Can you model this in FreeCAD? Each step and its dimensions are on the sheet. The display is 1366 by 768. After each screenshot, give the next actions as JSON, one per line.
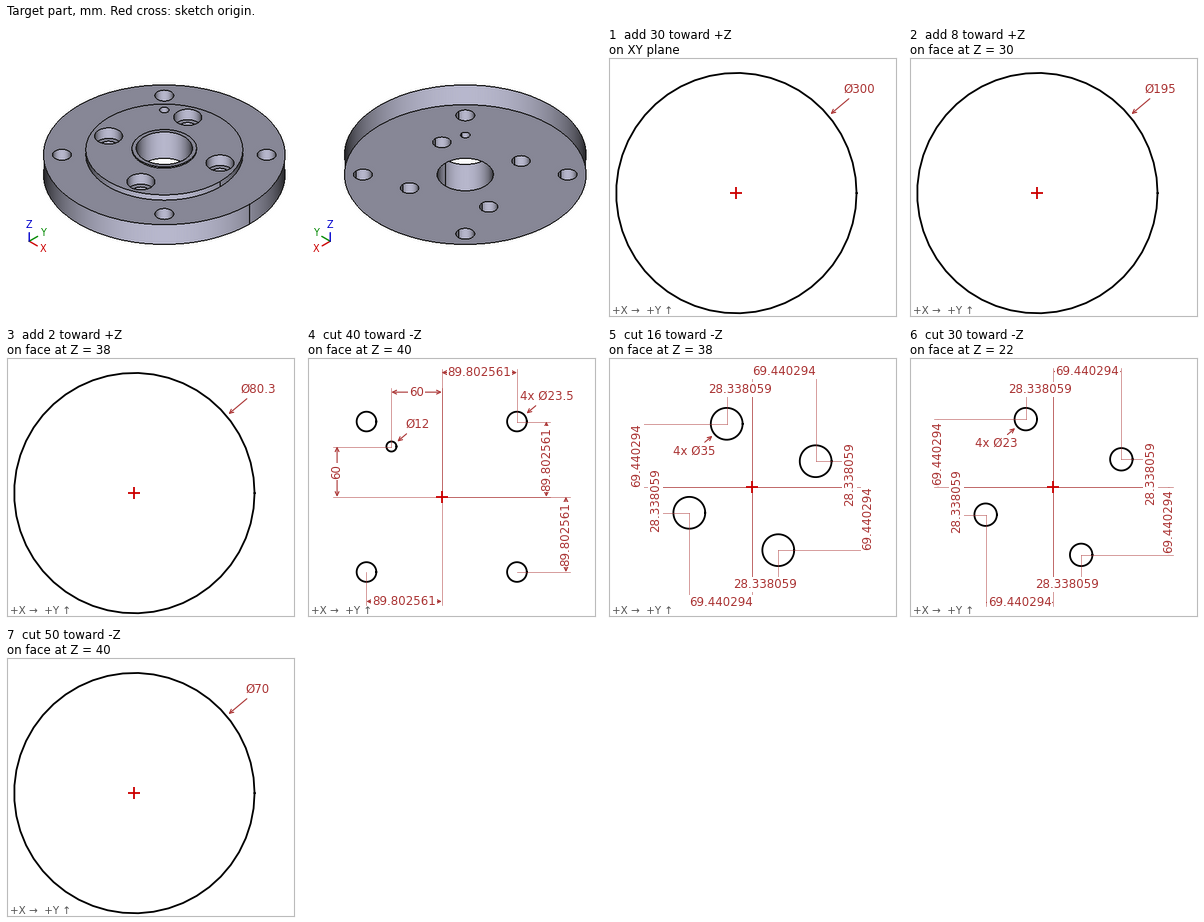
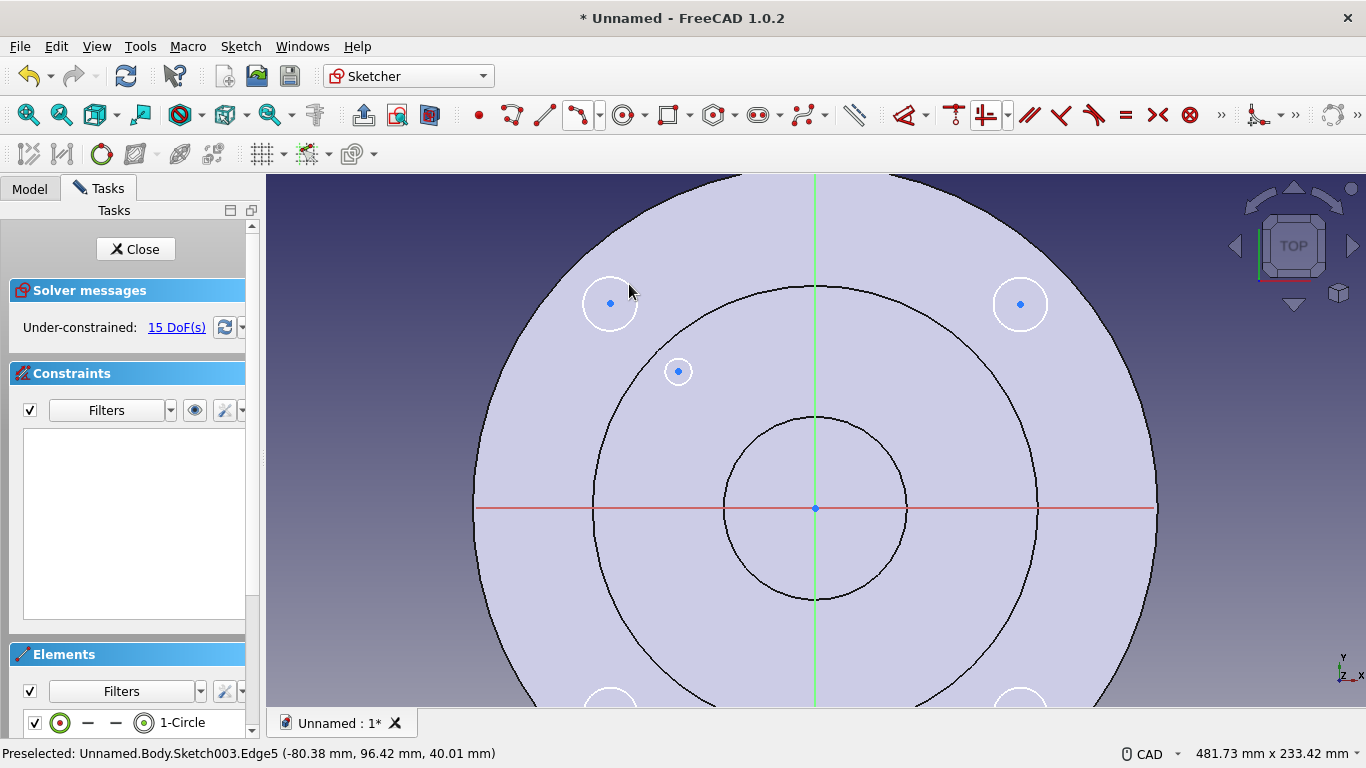
{"action": "left_click", "coordinate": [1039, 285]}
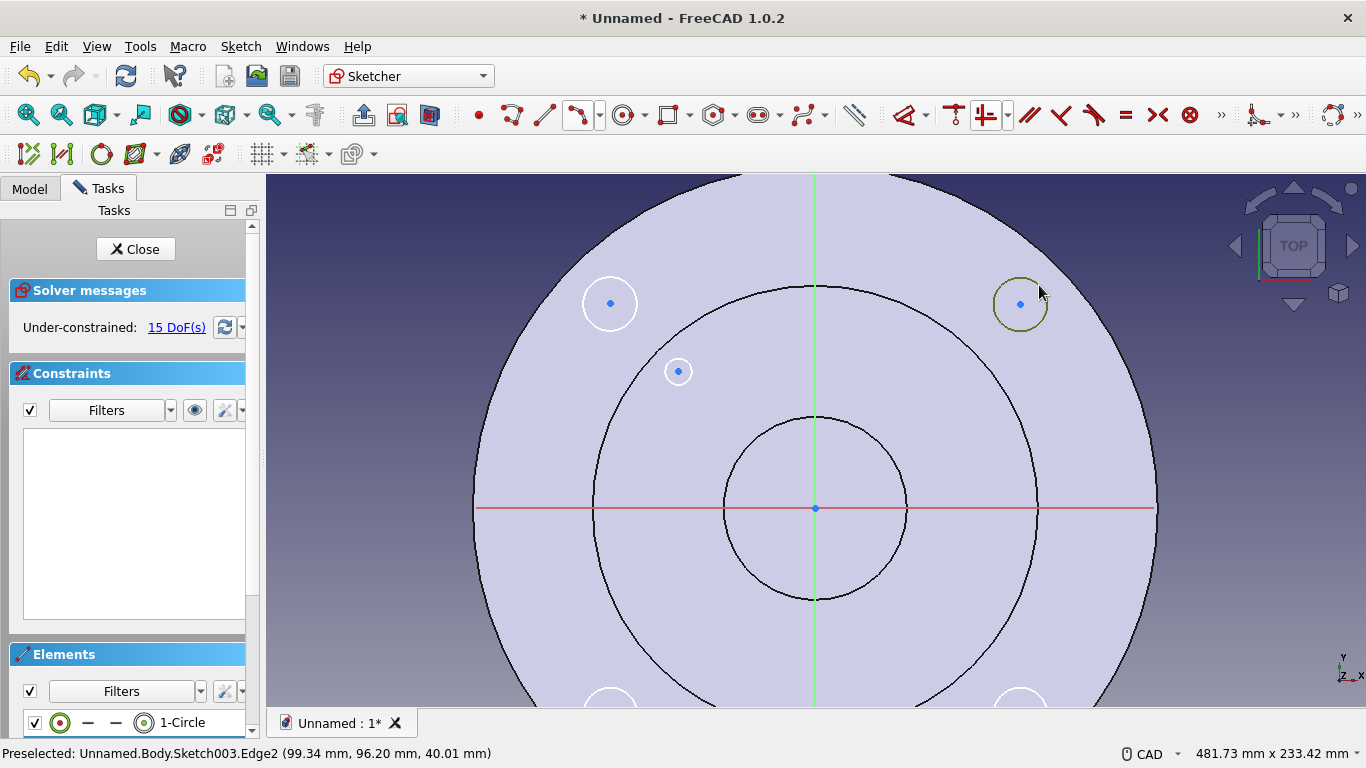
{"action": "scroll", "coordinate": [610, 303], "scroll_direction": "down", "scroll_amount": 2}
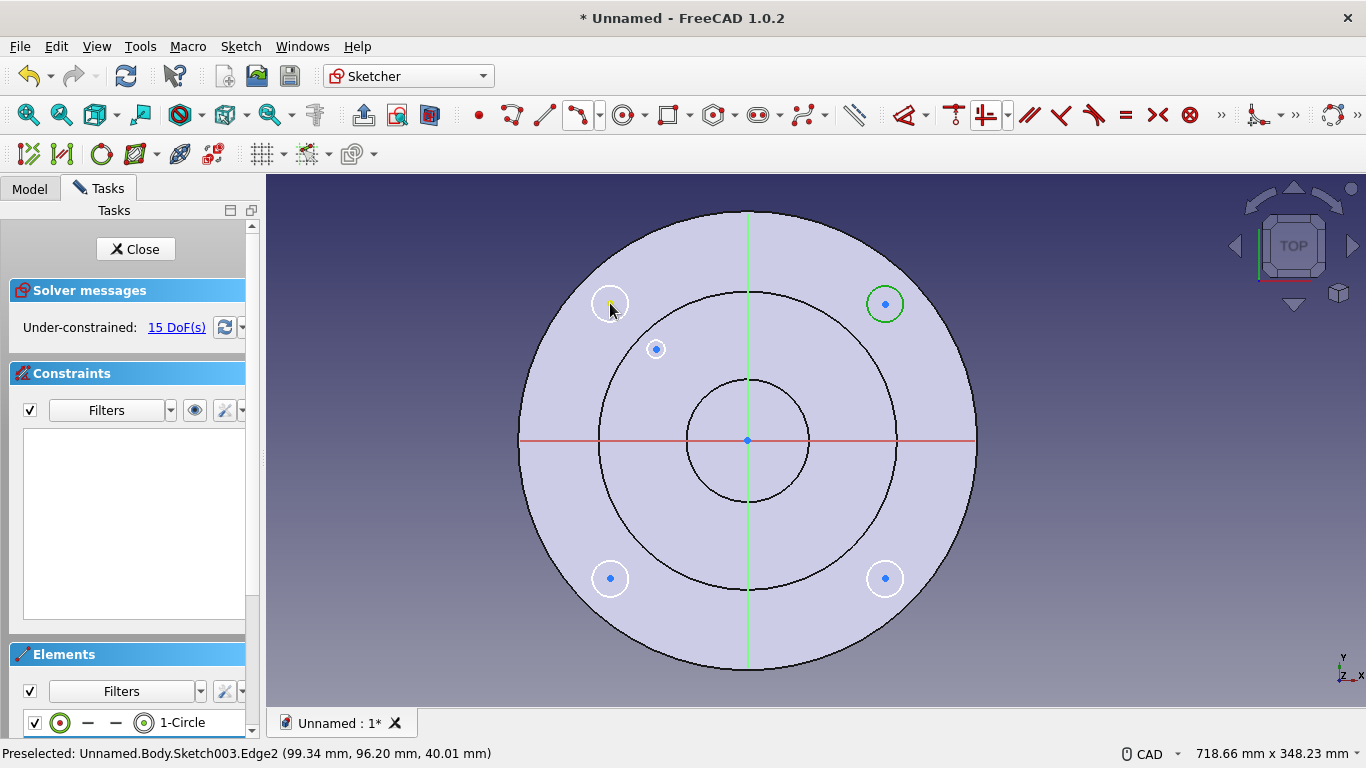
{"action": "left_click", "coordinate": [898, 566]}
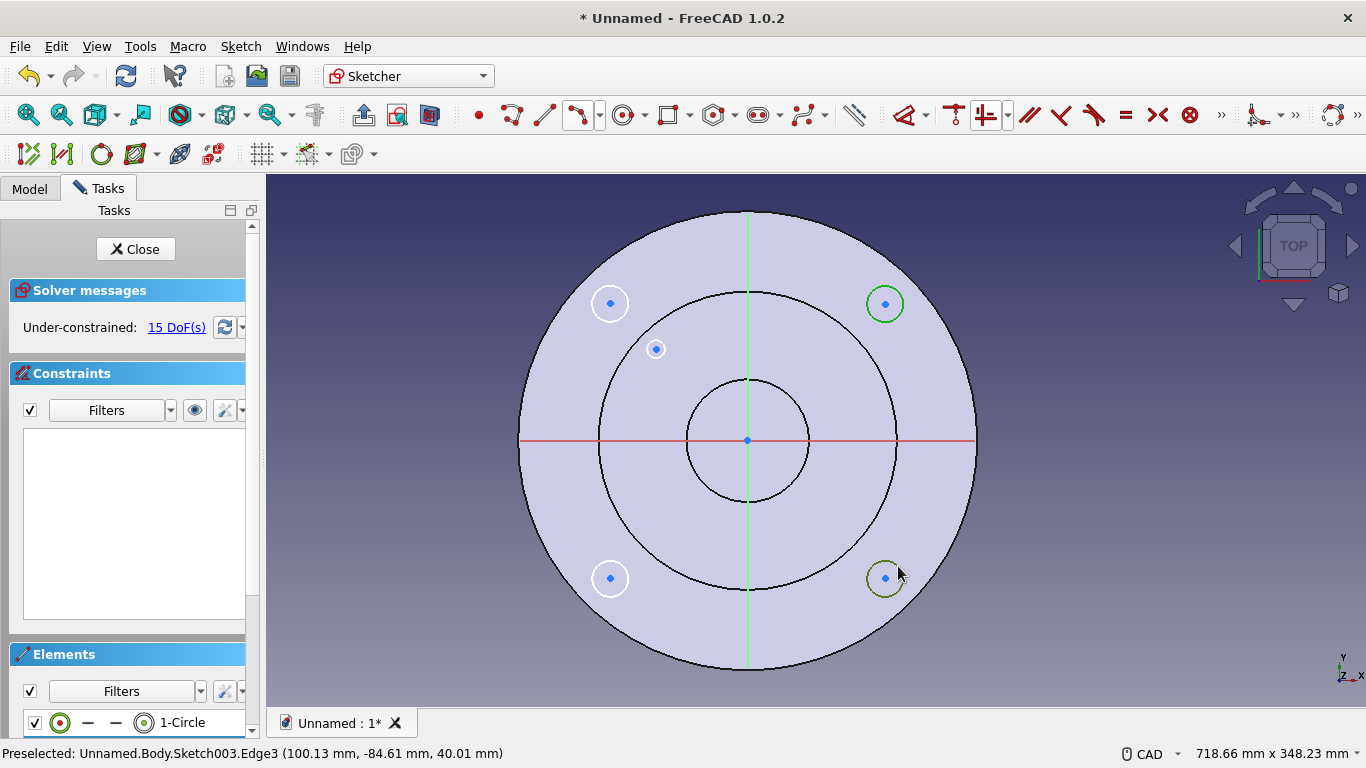
{"action": "left_click", "coordinate": [623, 566]}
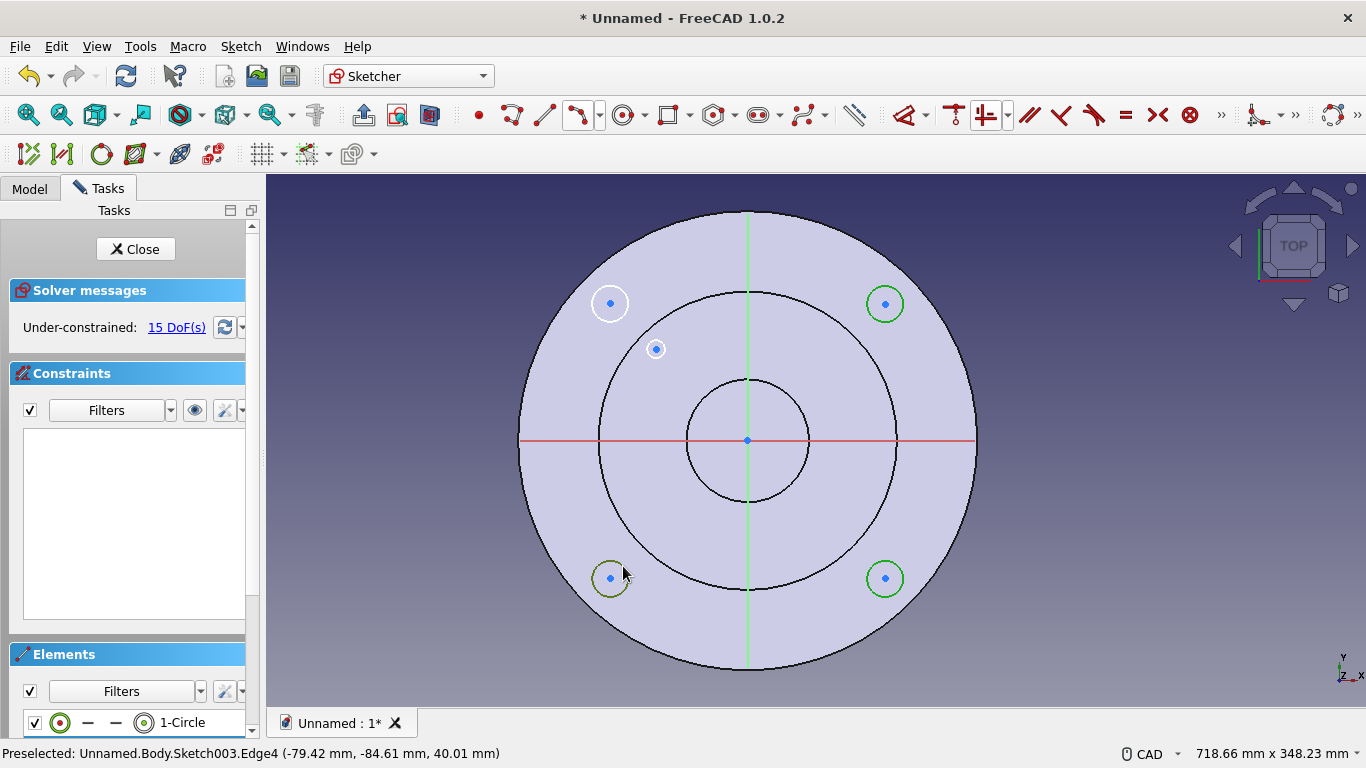
{"action": "left_click", "coordinate": [623, 291]}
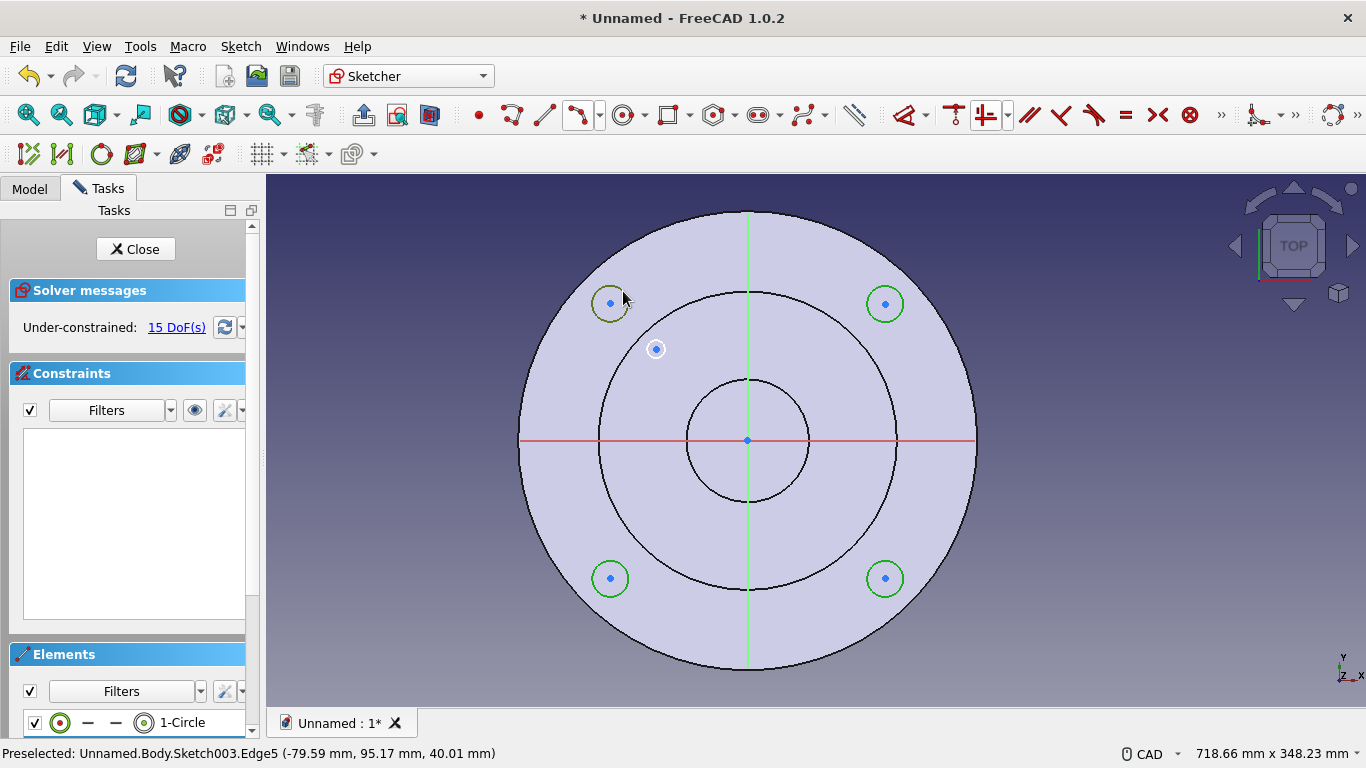
{"action": "left_click", "coordinate": [1126, 116]}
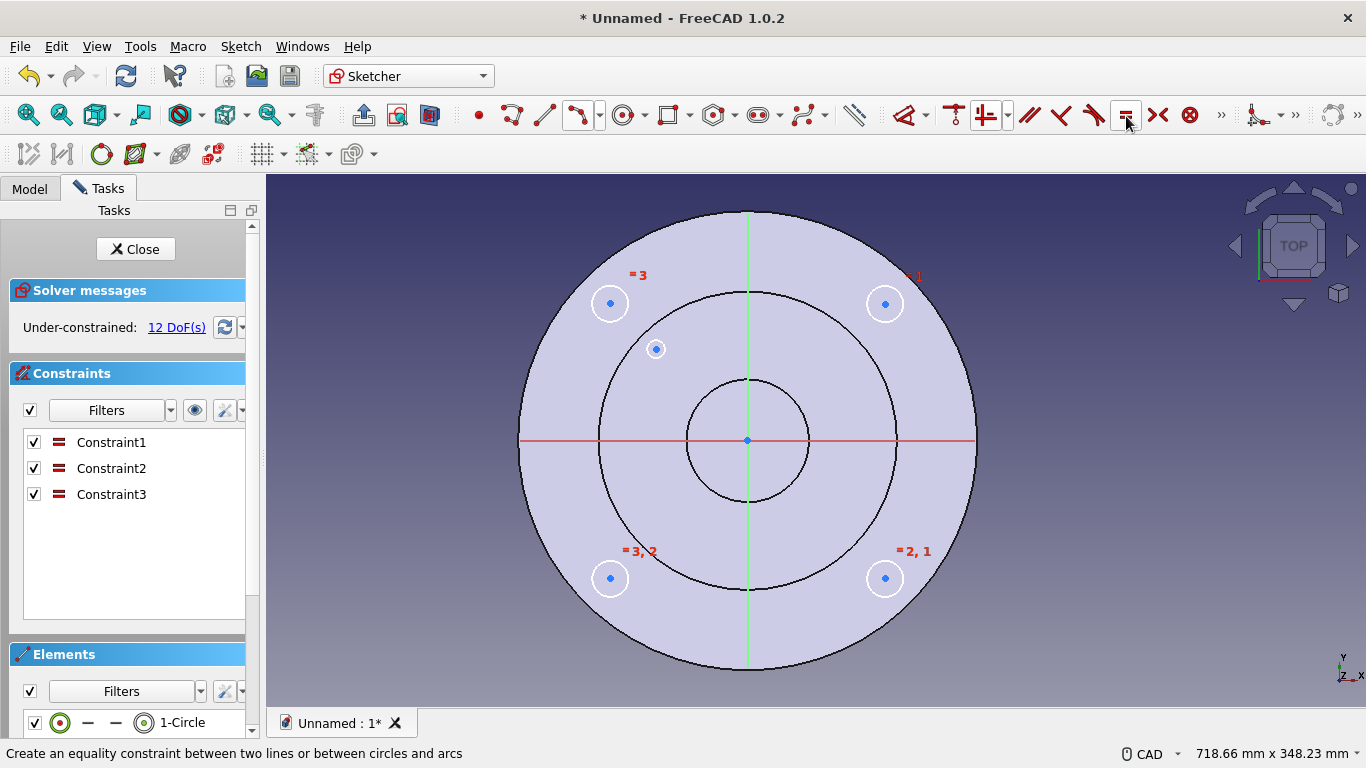
{"action": "left_click", "coordinate": [885, 304]}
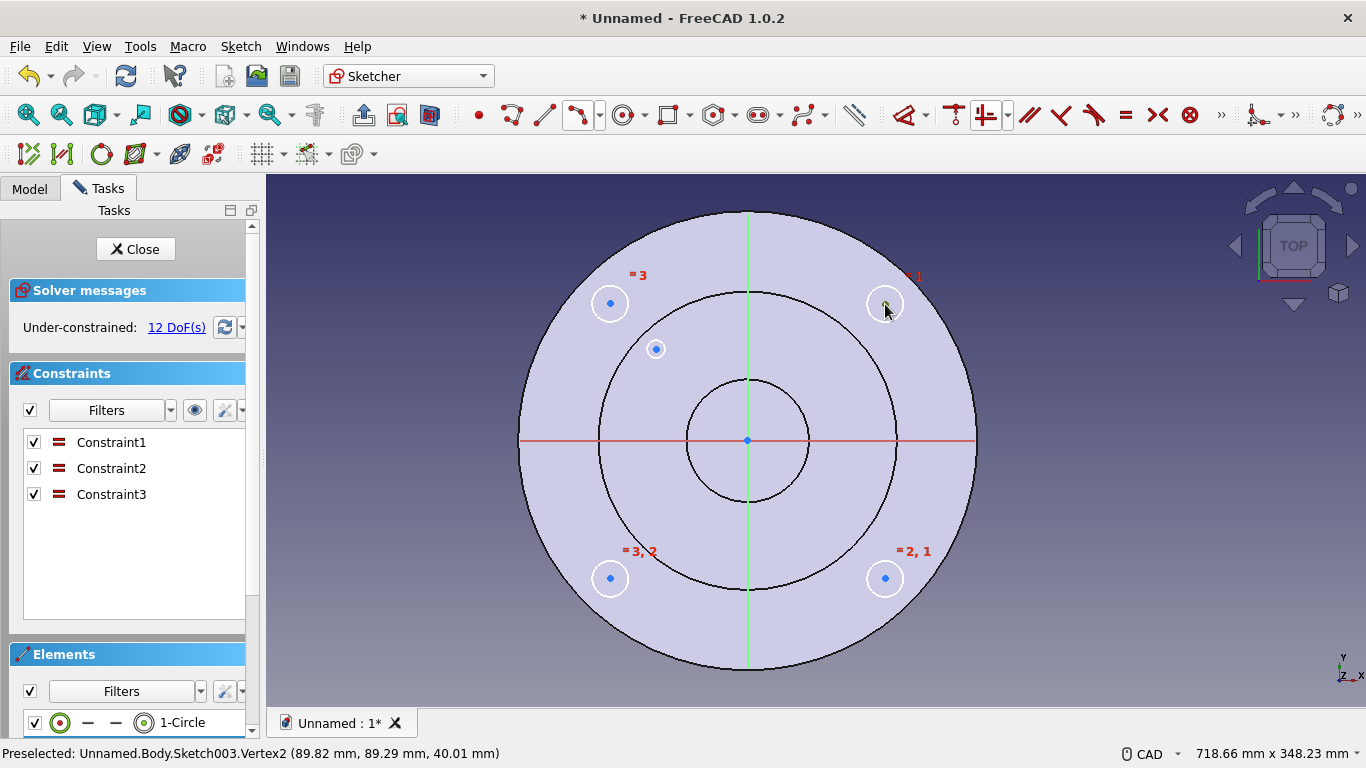
{"action": "left_click", "coordinate": [885, 579]}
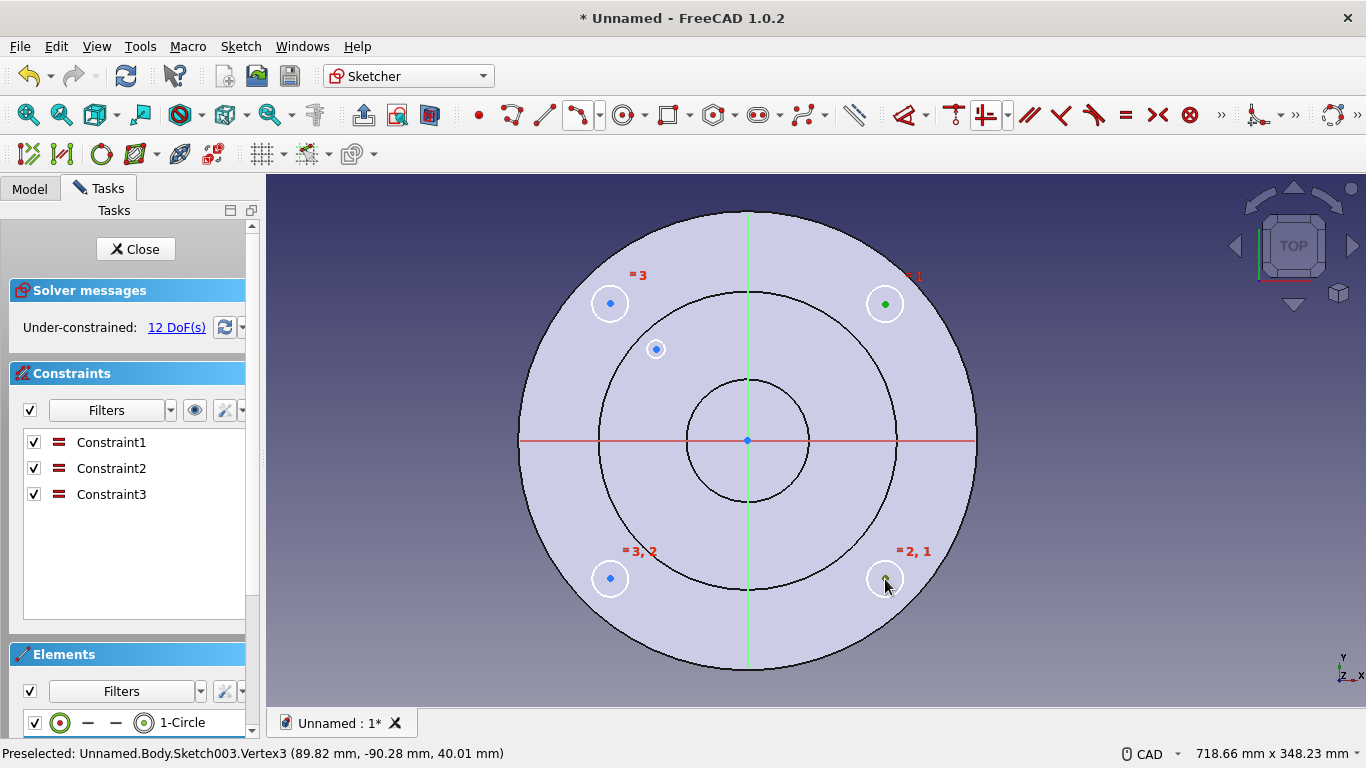
{"action": "left_click", "coordinate": [1008, 116]}